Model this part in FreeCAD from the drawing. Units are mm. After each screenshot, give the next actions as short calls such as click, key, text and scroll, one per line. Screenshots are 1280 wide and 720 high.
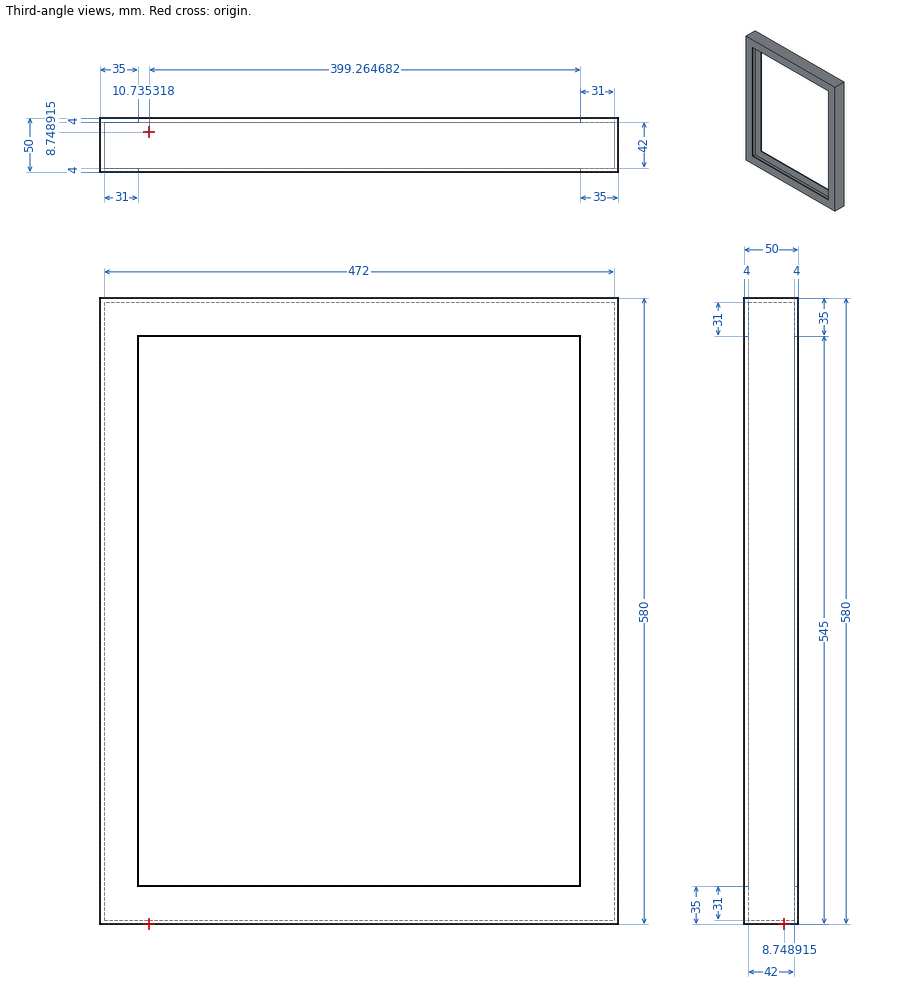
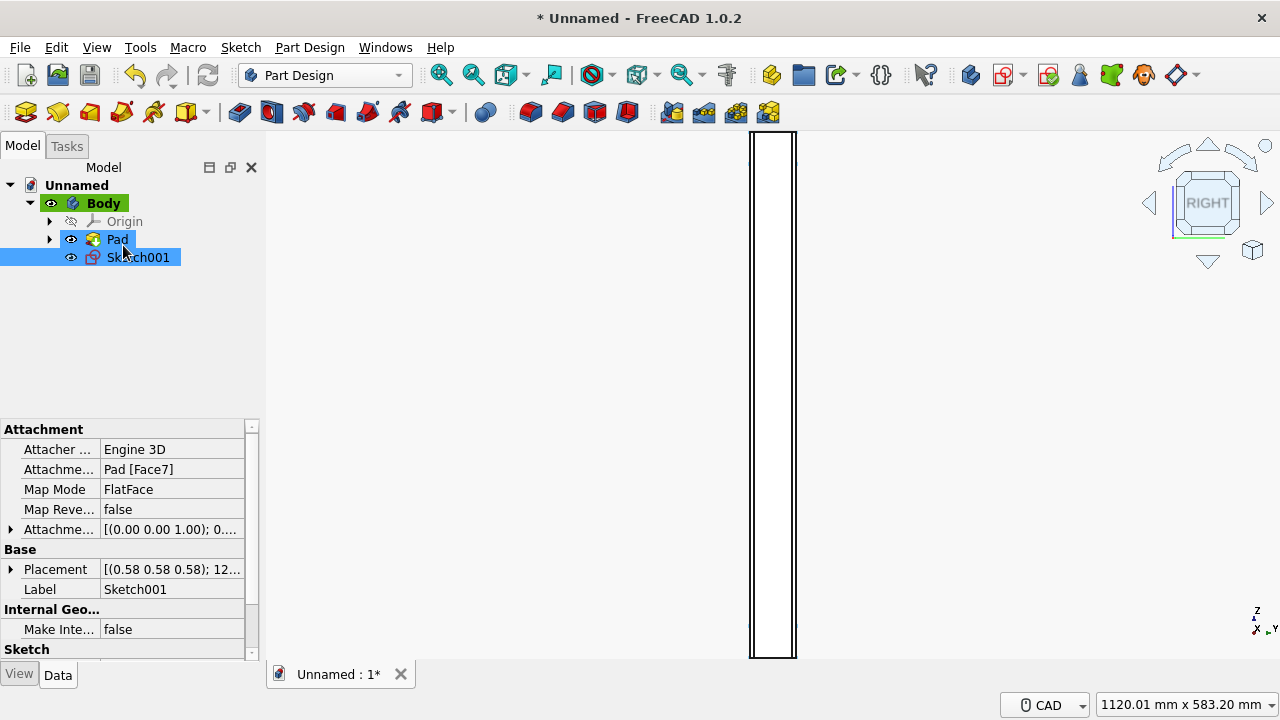
click(26, 112)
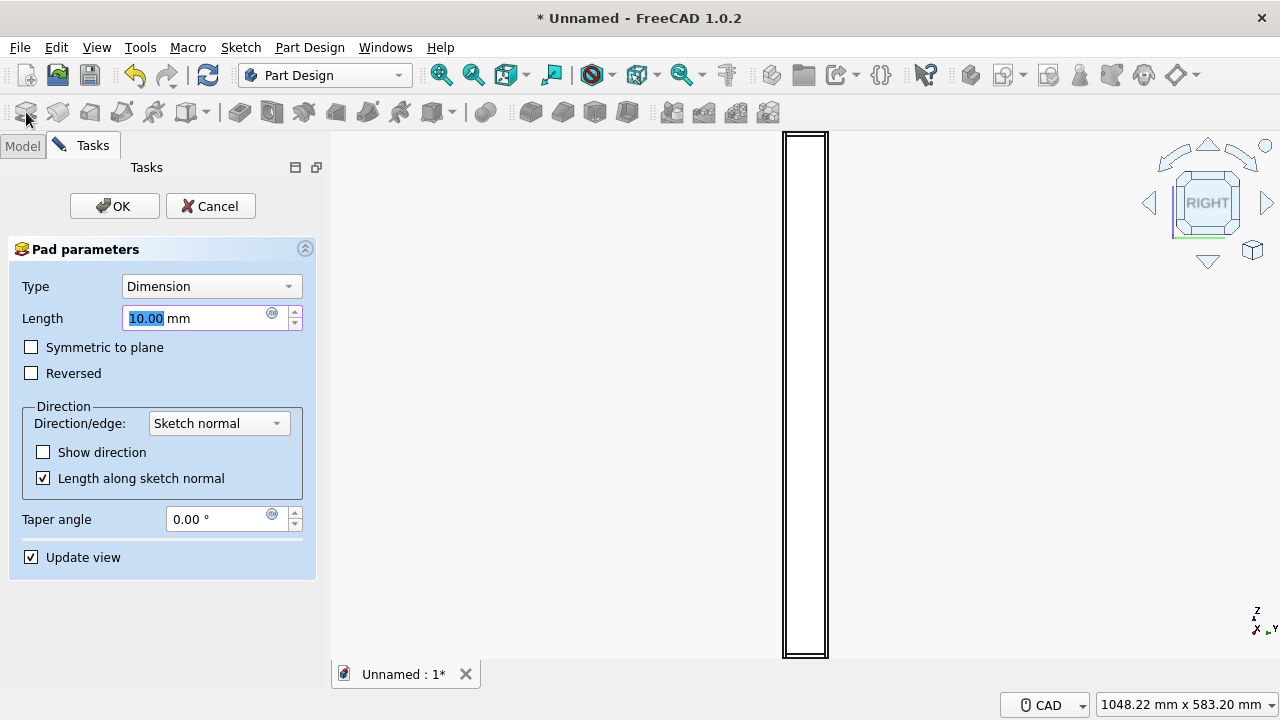
text(472)
key(Tab)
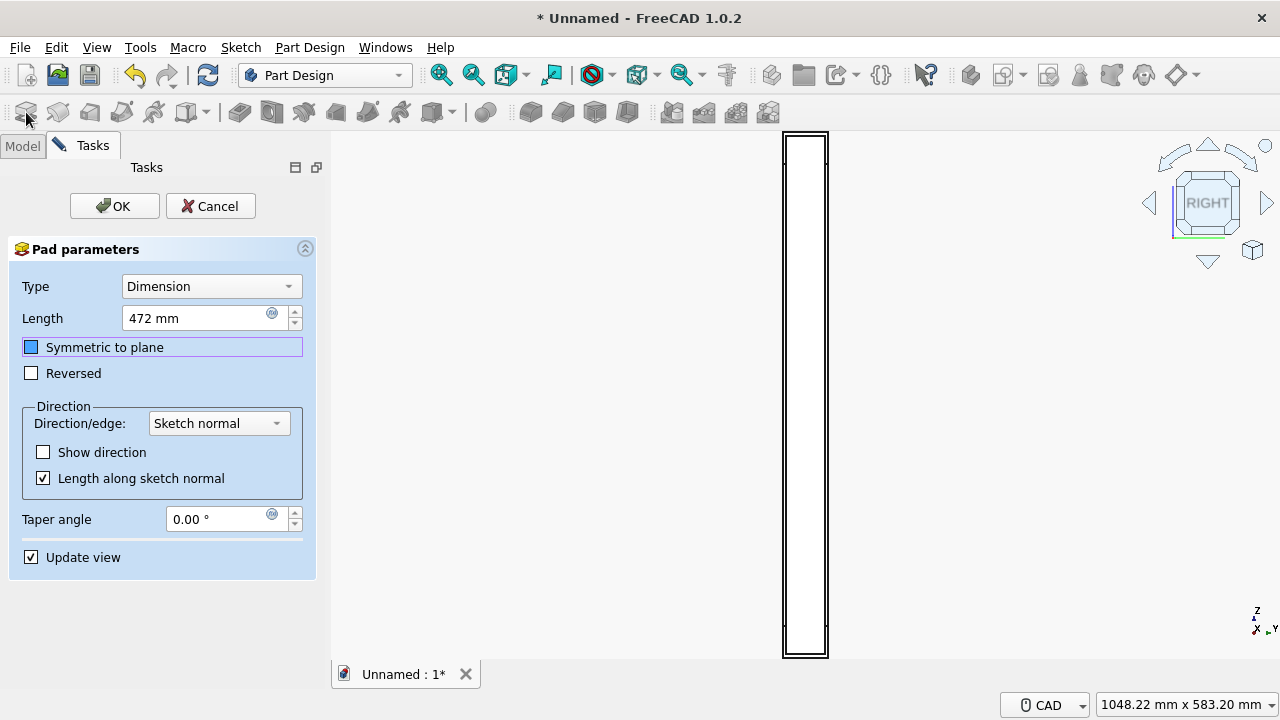
click(115, 206)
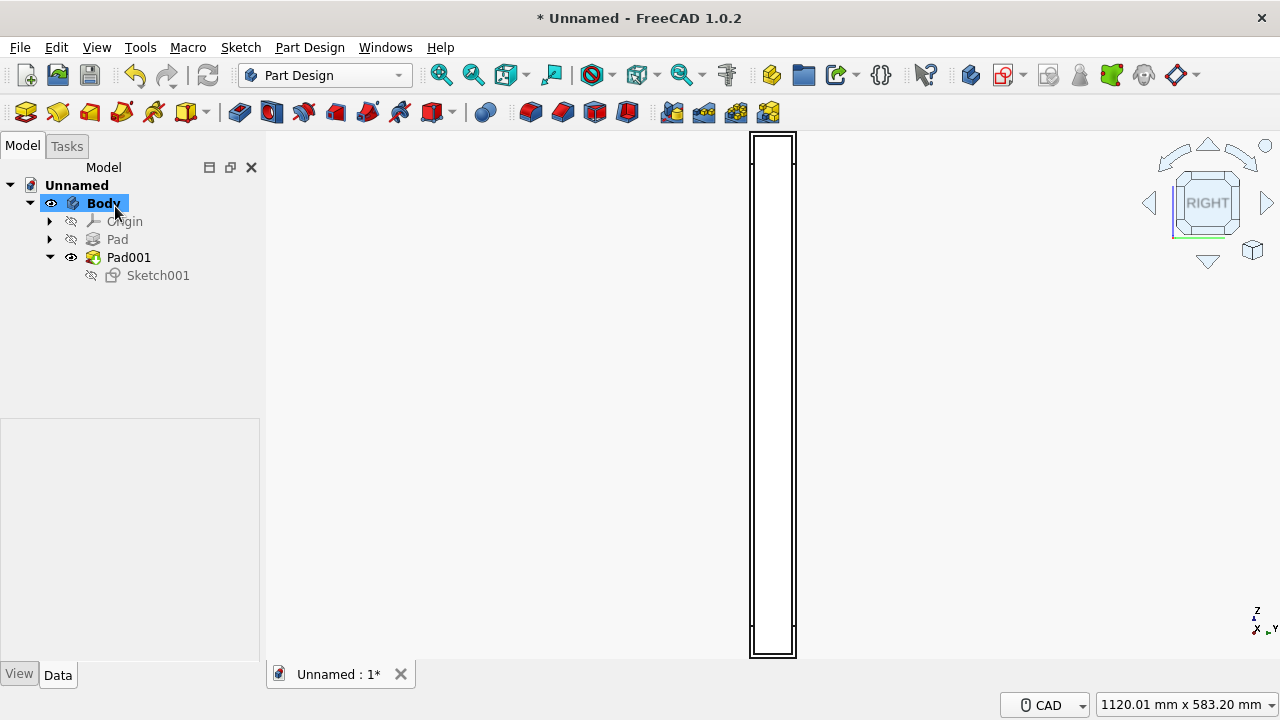
key(0)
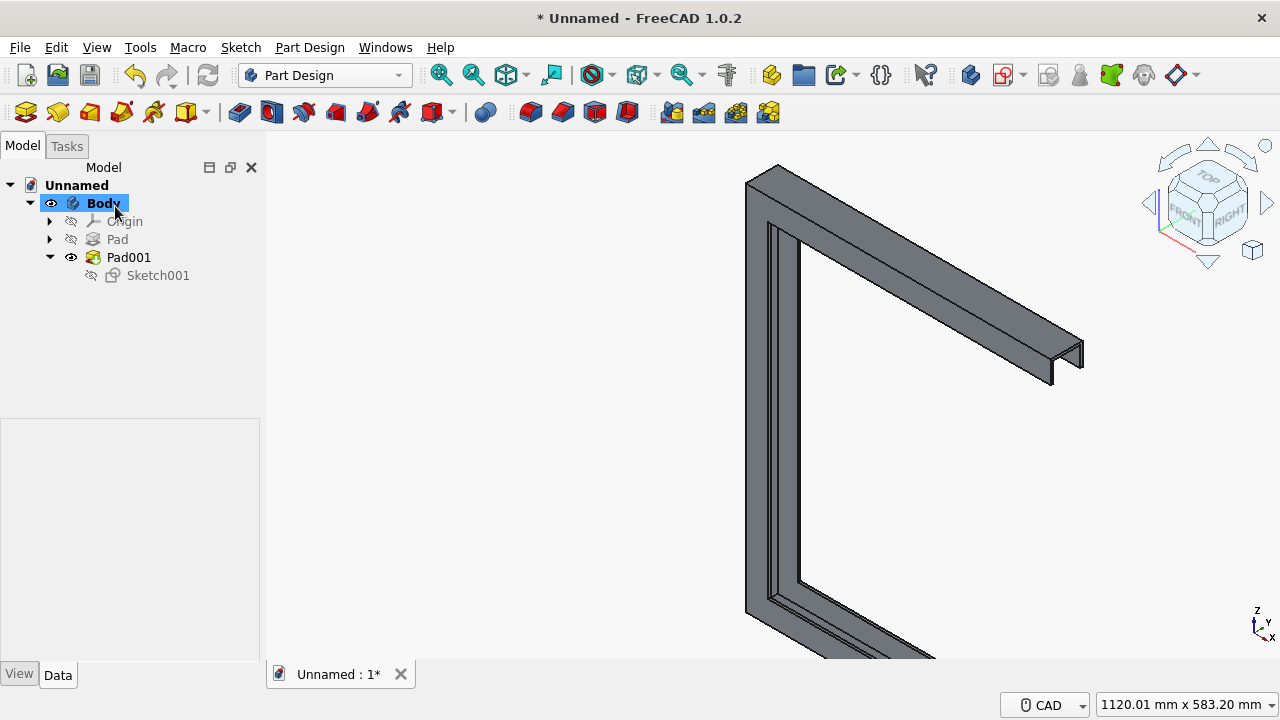
key(v)
key(f)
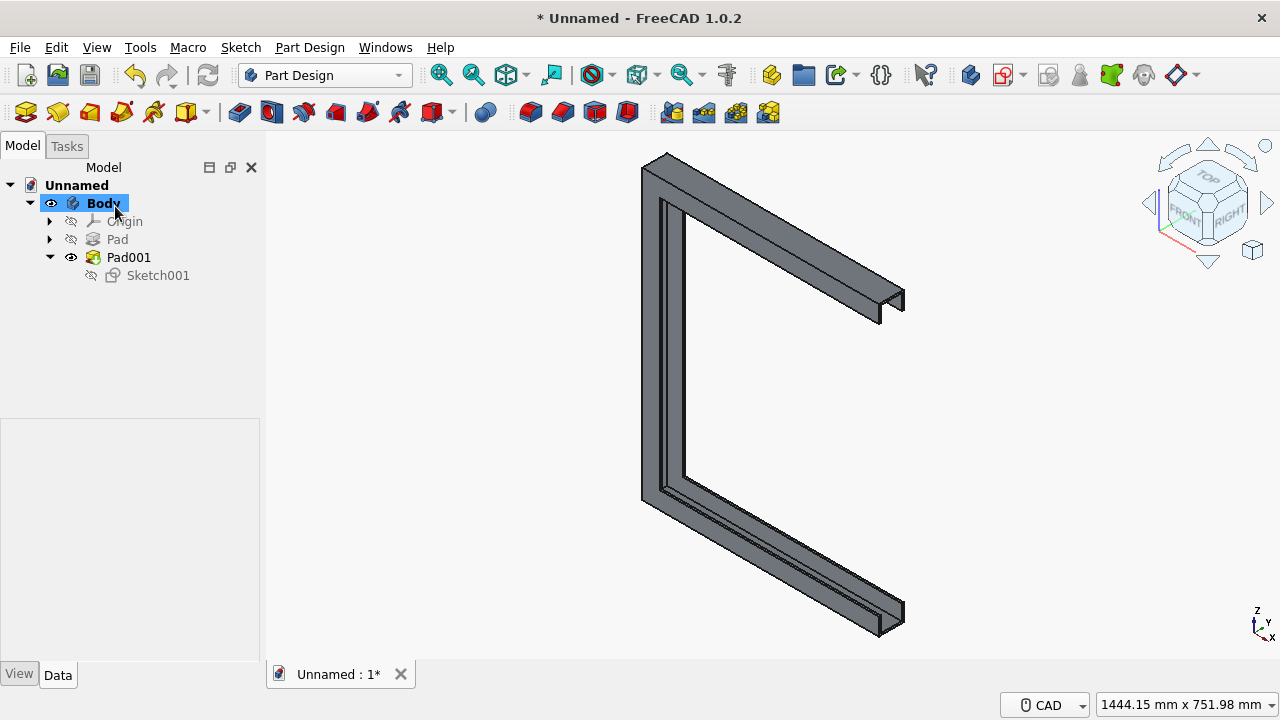
click(874, 286)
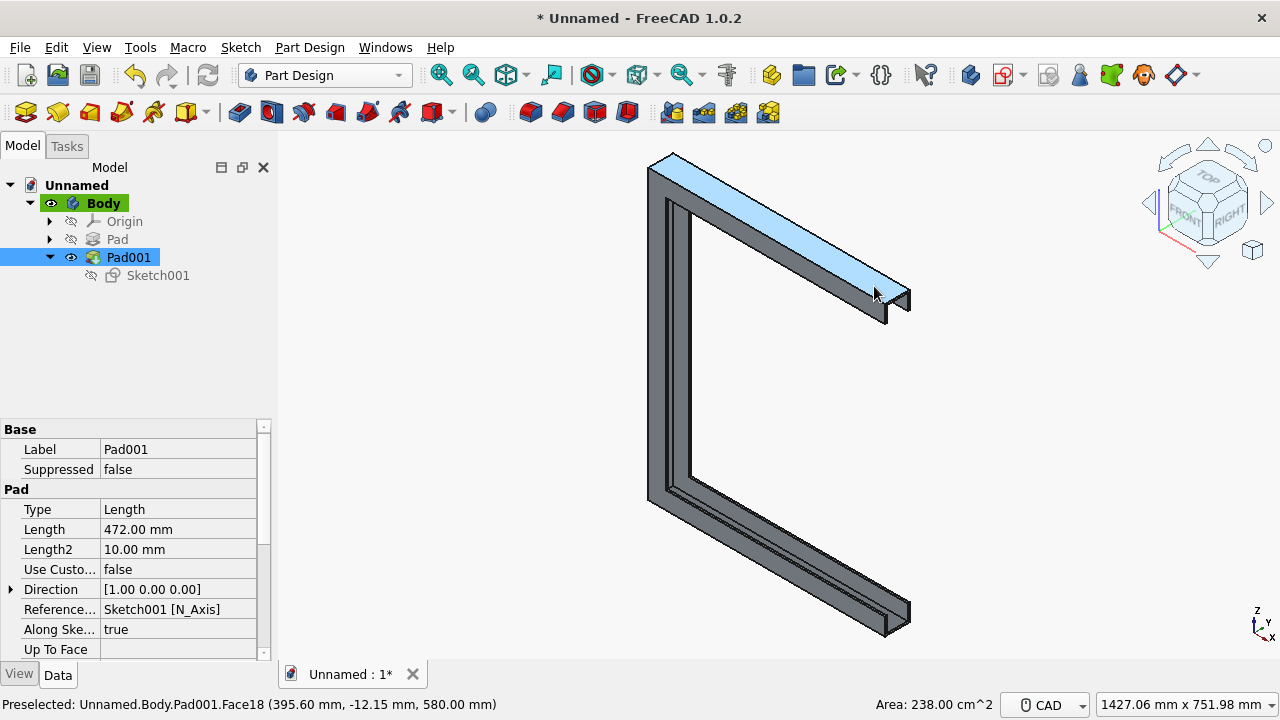
click(1004, 76)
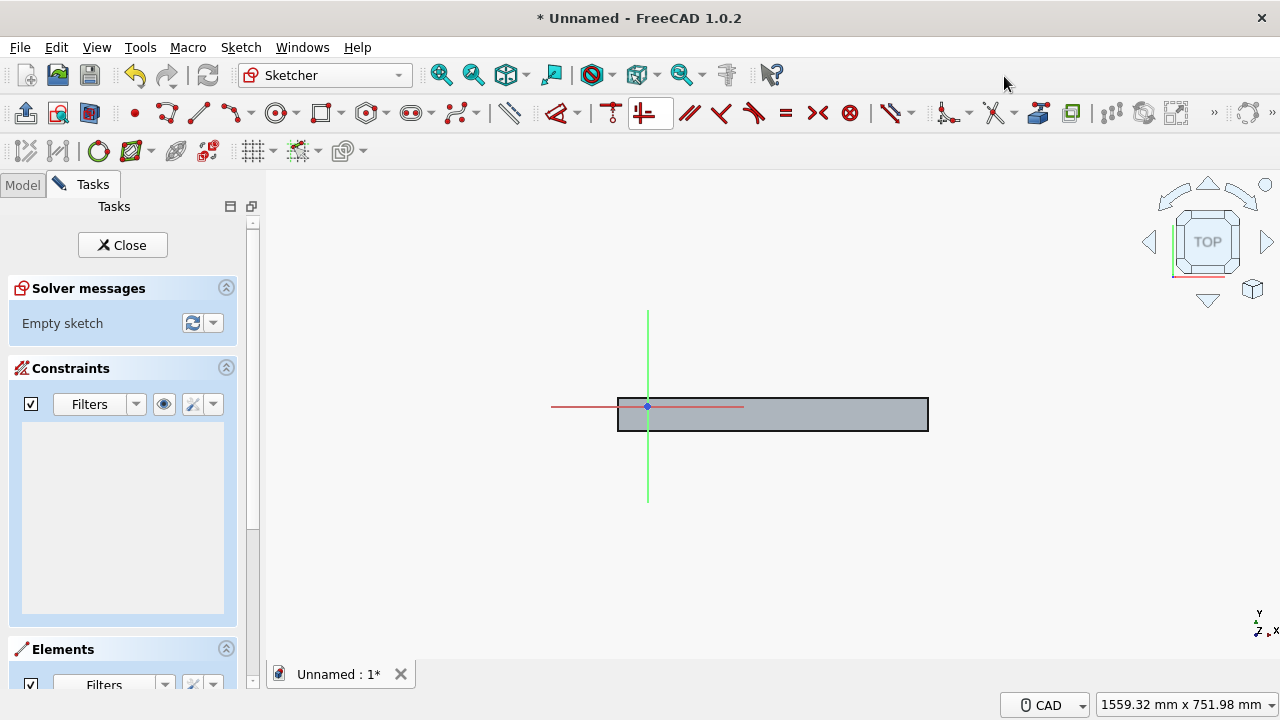
scroll(946, 415, up, 11)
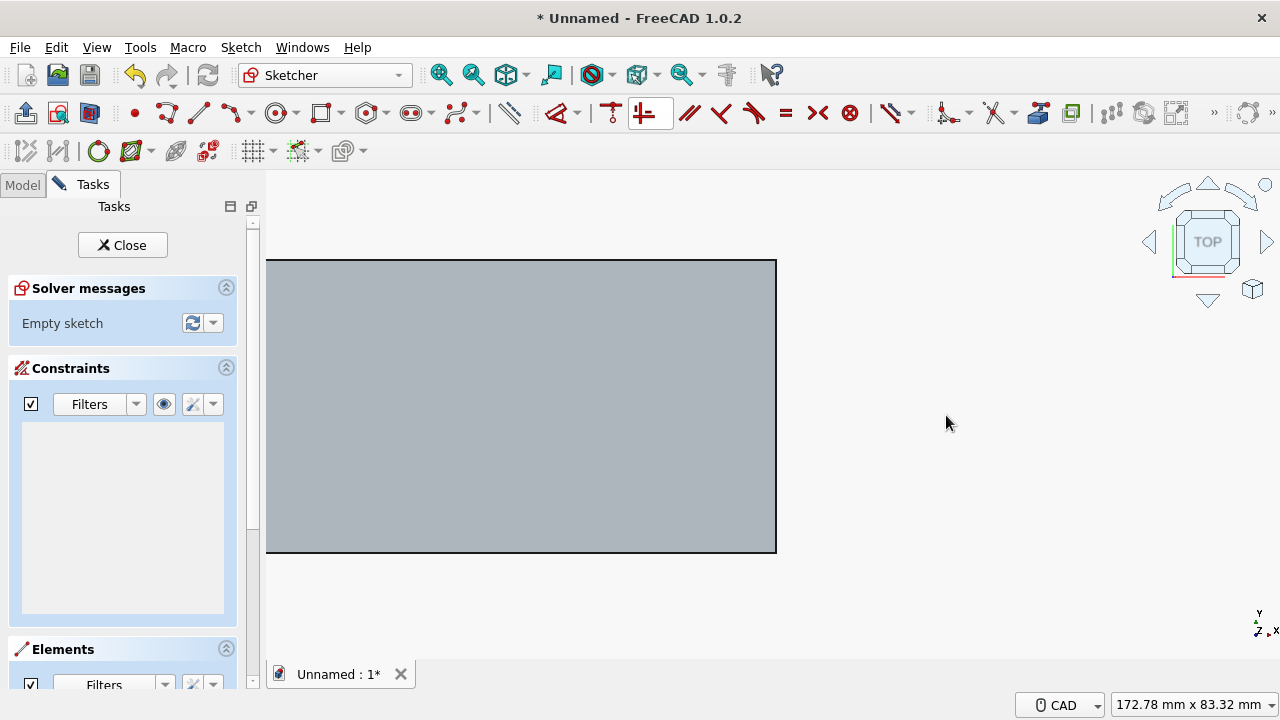
click(168, 114)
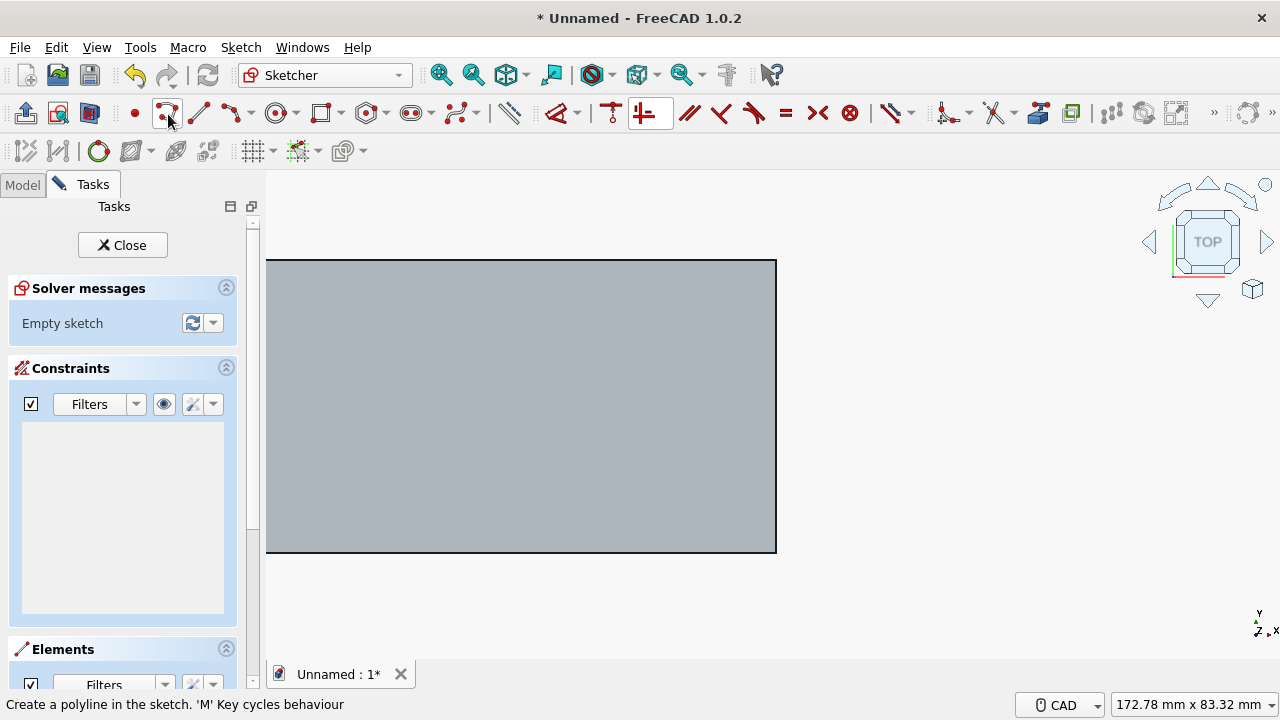
click(594, 283)
click(776, 283)
click(776, 530)
click(594, 530)
click(594, 553)
click(800, 553)
click(800, 260)
click(594, 260)
click(594, 284)
key(Escape)
key(Escape)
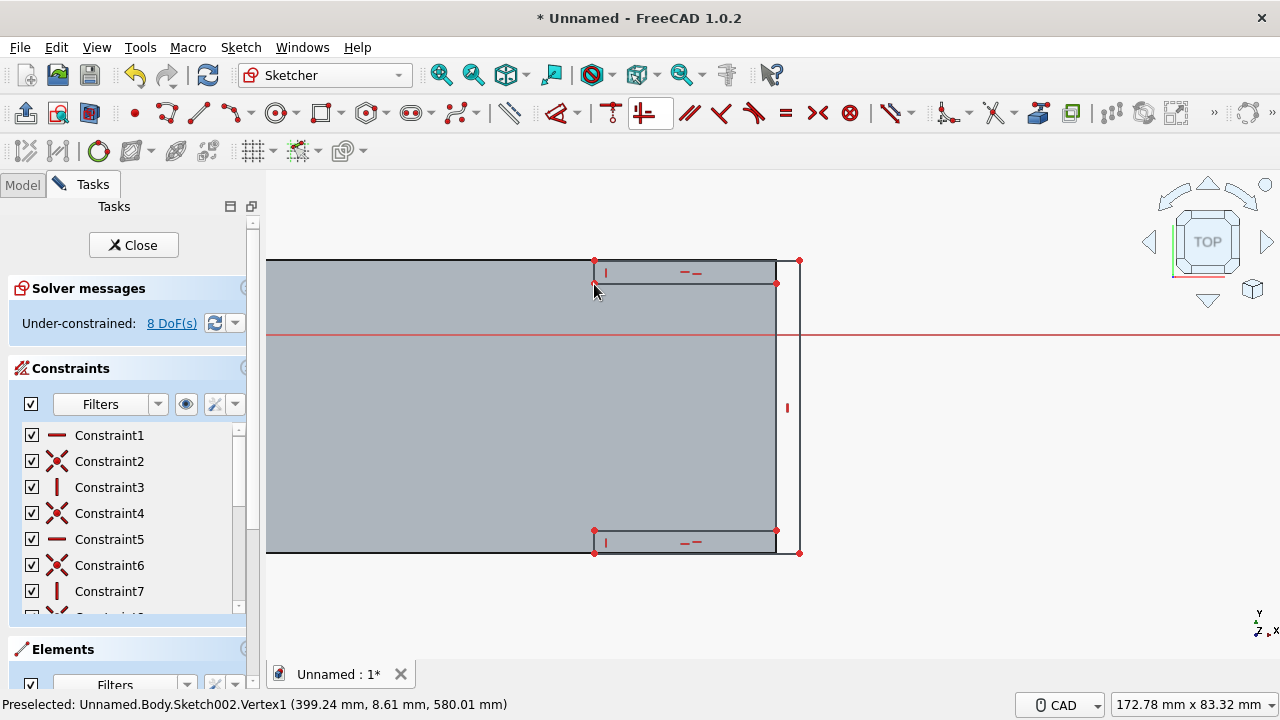
click(556, 114)